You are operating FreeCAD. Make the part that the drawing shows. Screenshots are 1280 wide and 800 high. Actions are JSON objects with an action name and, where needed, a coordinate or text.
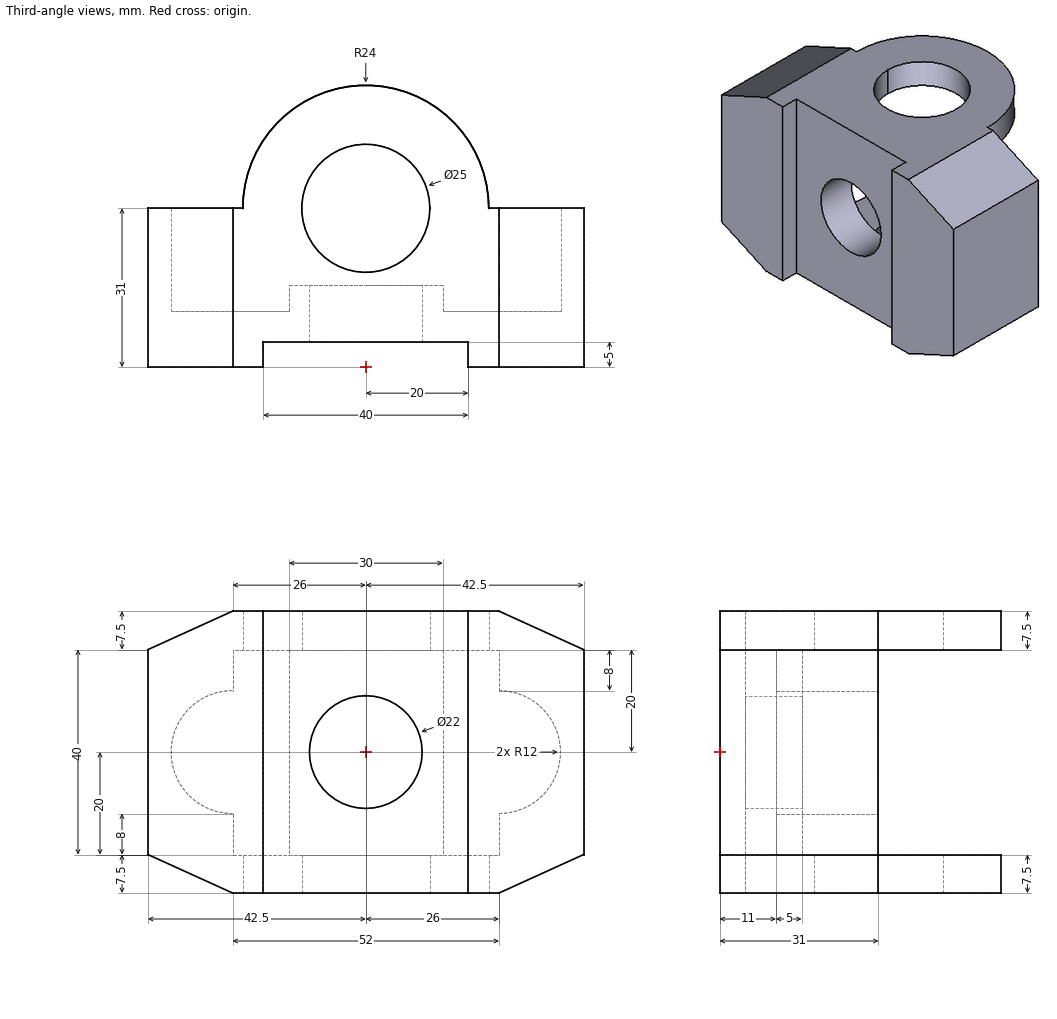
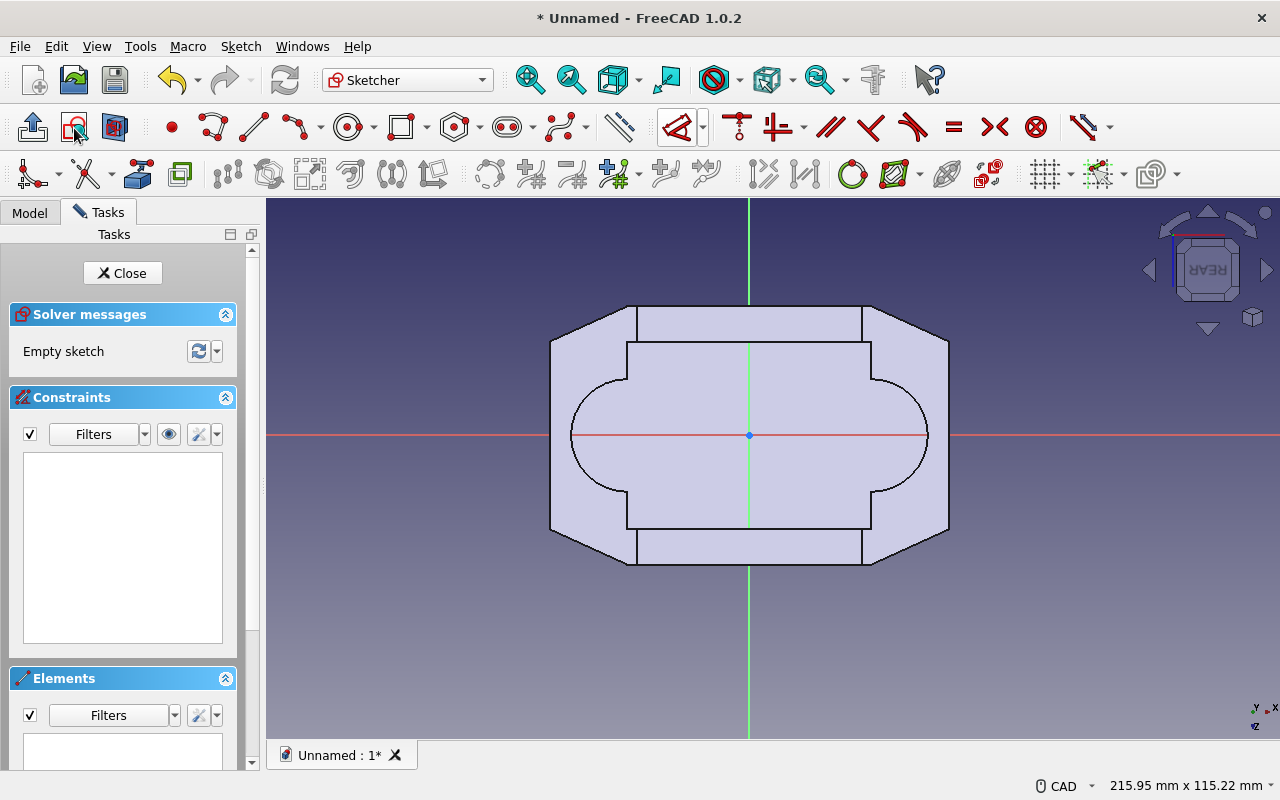
{"action": "left_click", "coordinate": [115, 128]}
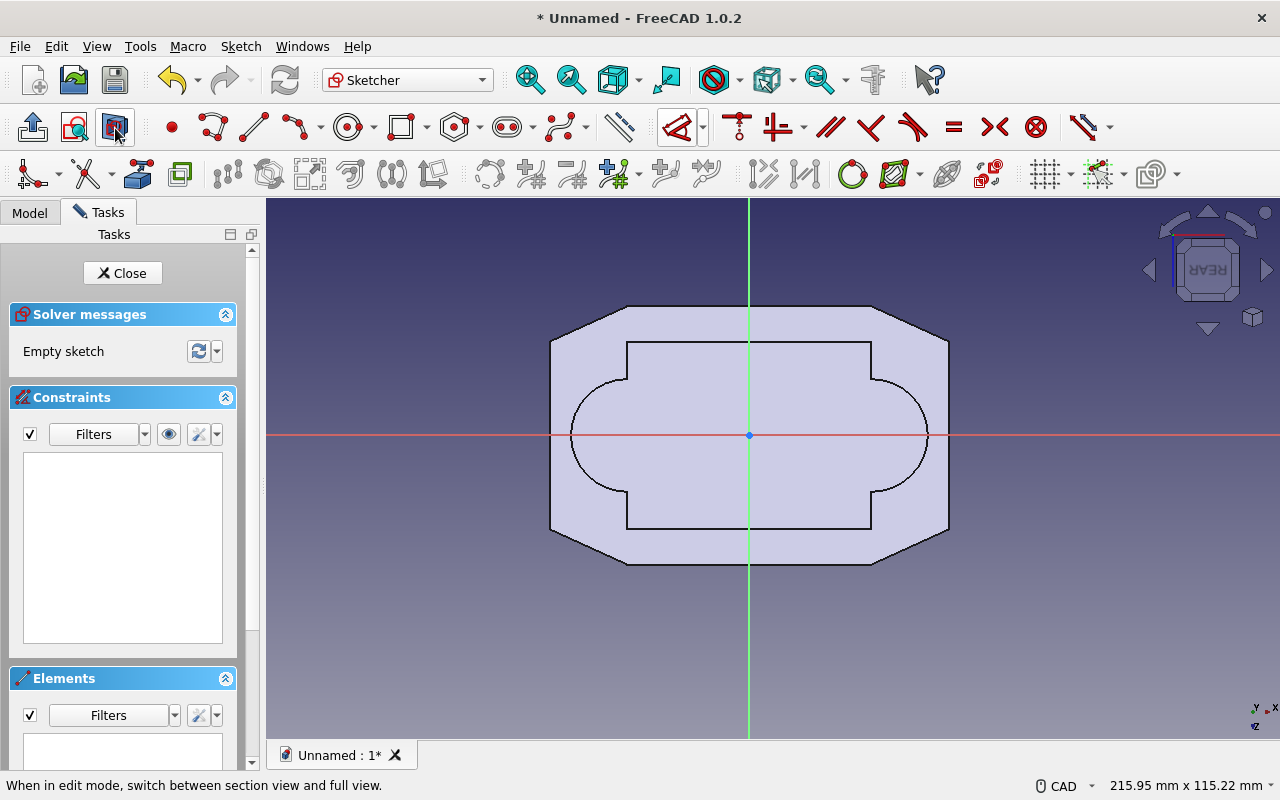
{"action": "scroll", "coordinate": [804, 395], "scroll_direction": "up", "scroll_amount": 3}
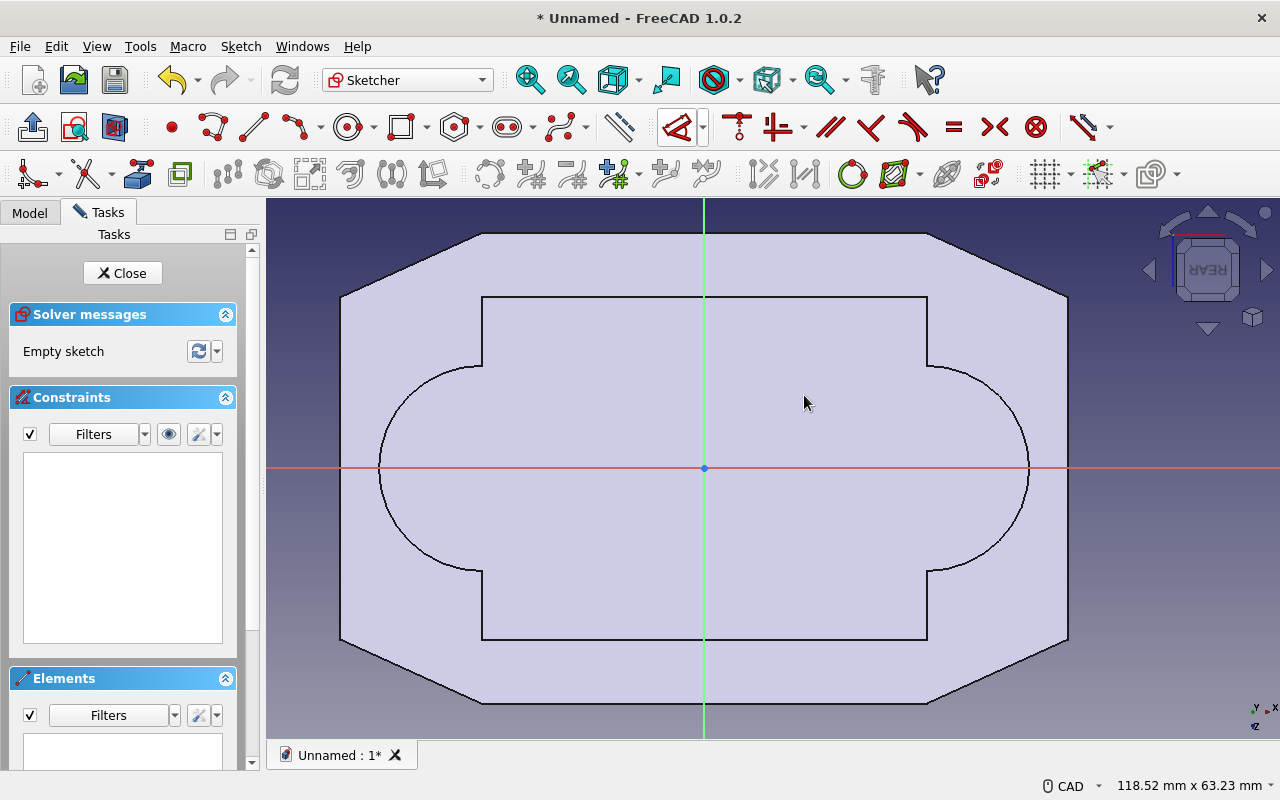
{"action": "key", "text": "g v"}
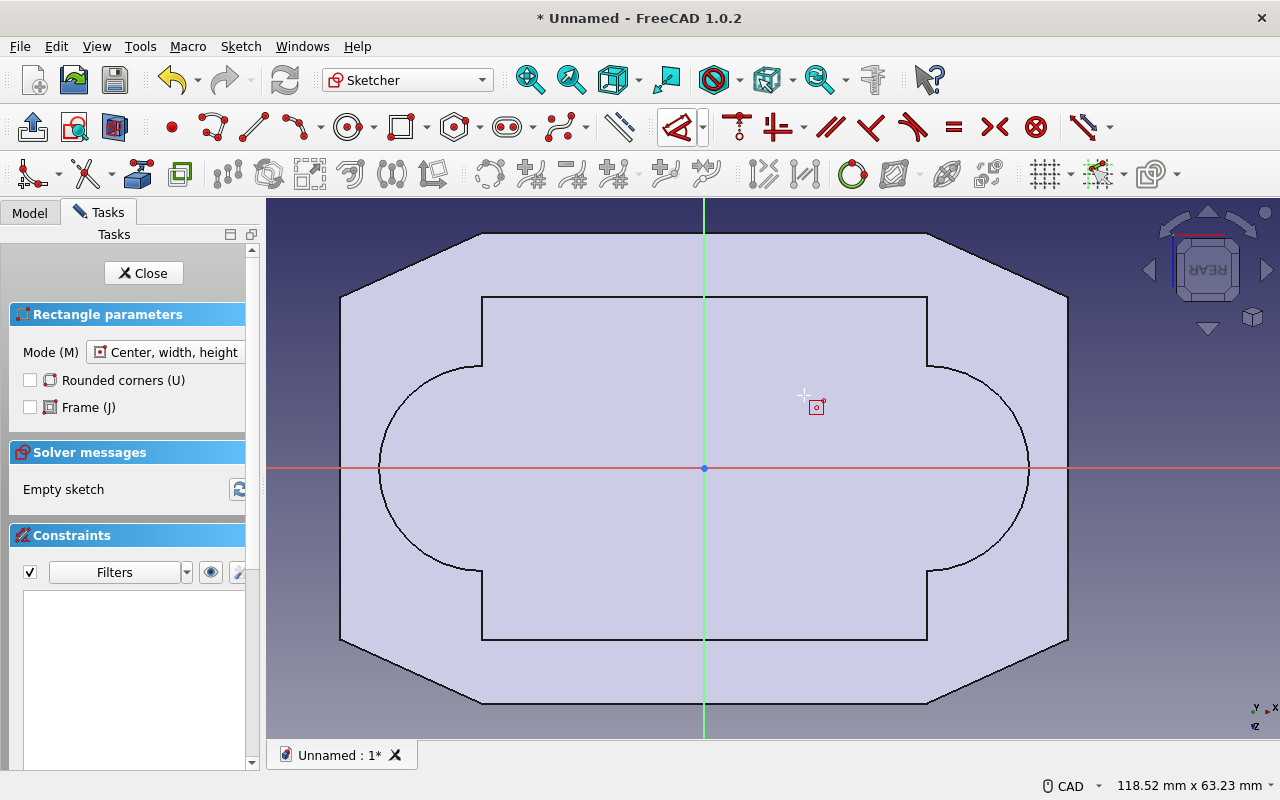
{"action": "left_click", "coordinate": [704, 468]}
{"action": "left_click", "coordinate": [832, 297]}
{"action": "key", "text": "Escape"}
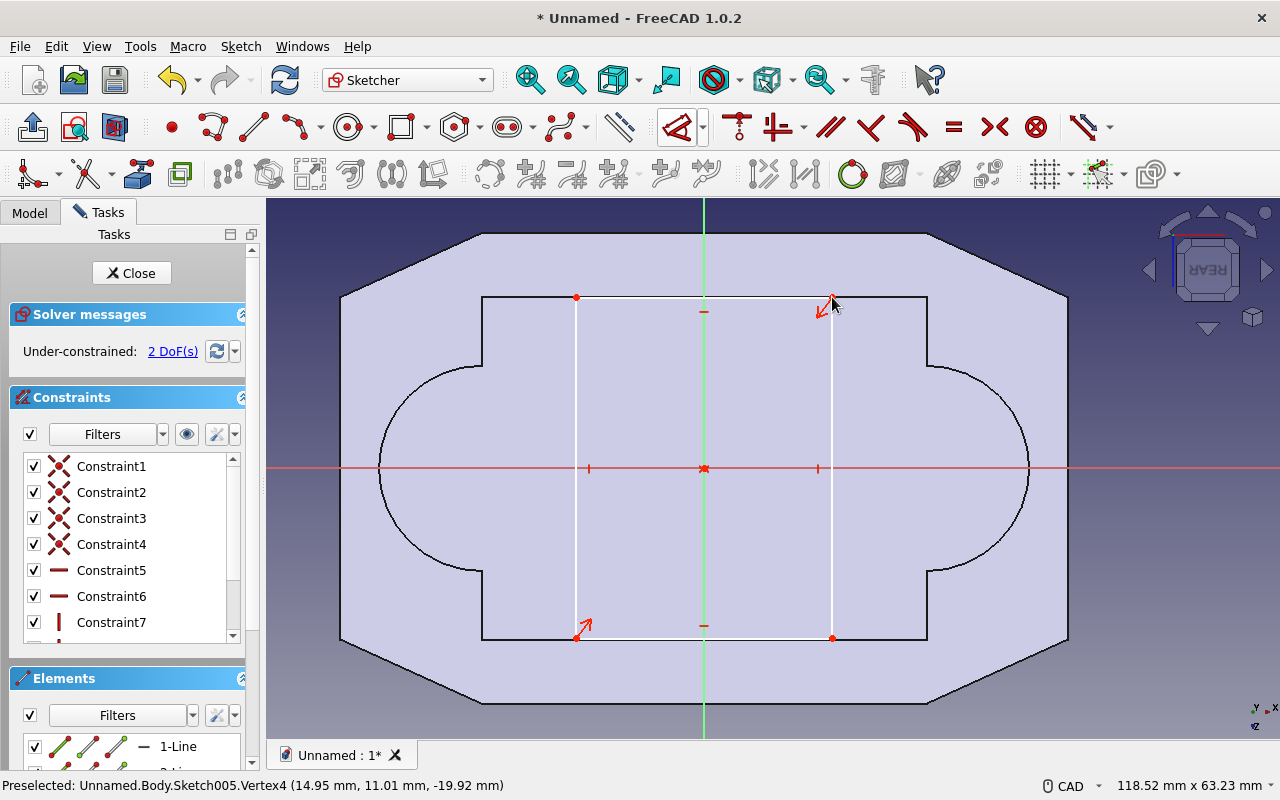
{"action": "left_click", "coordinate": [653, 639]}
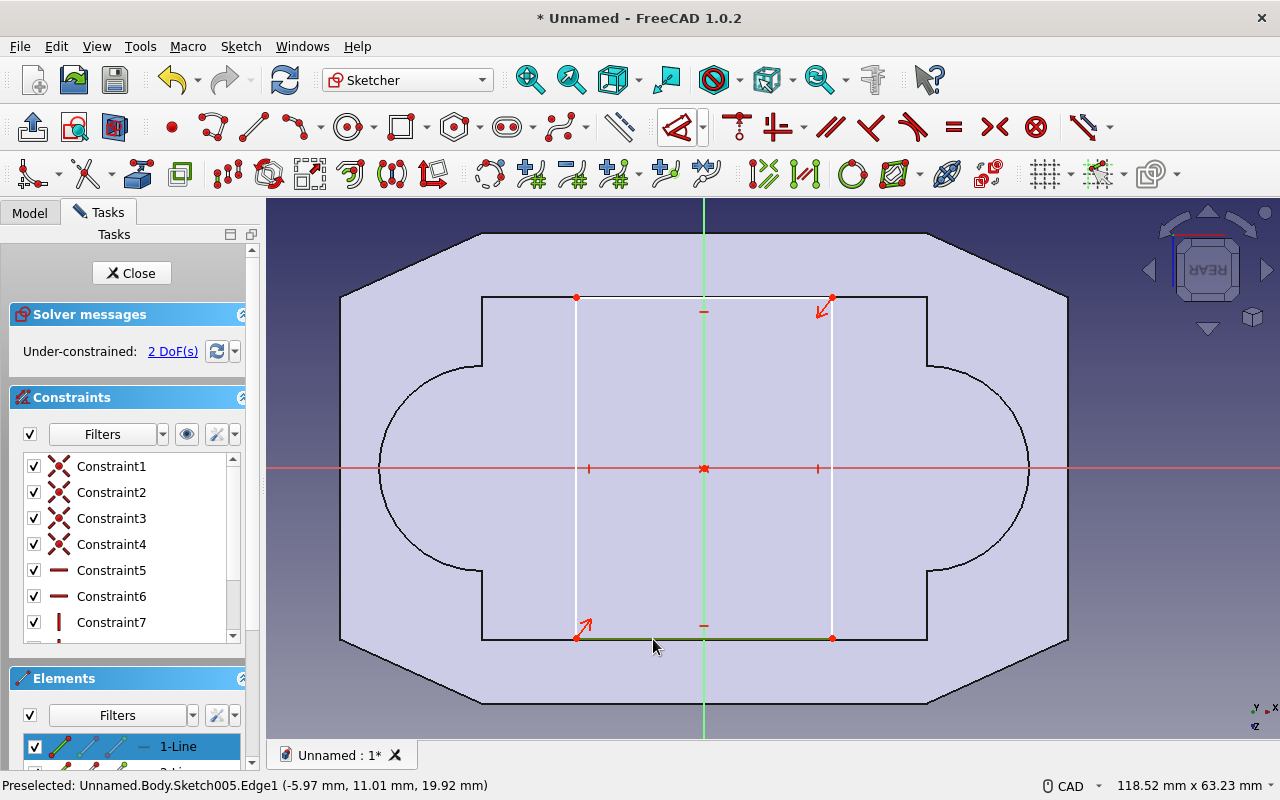
{"action": "key", "text": "l"}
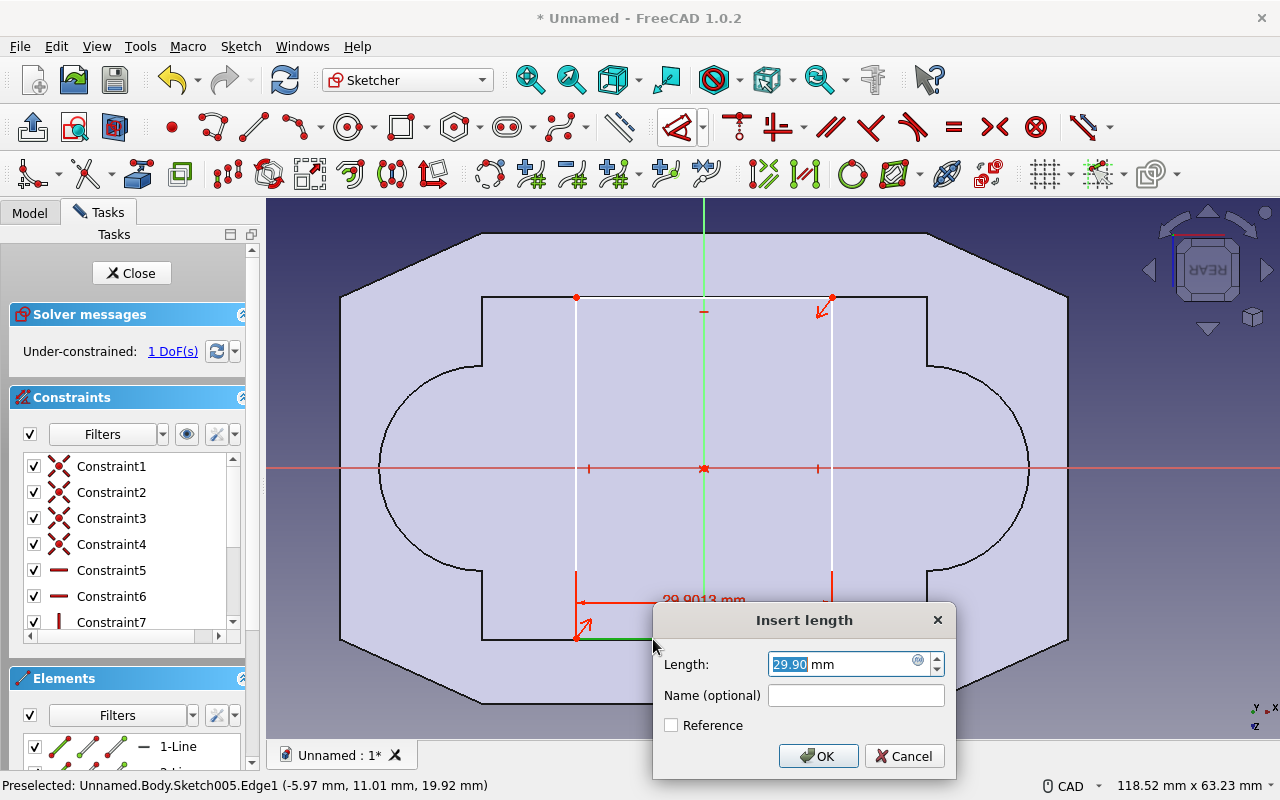
{"action": "type", "text": "30"}
{"action": "key", "text": "Return"}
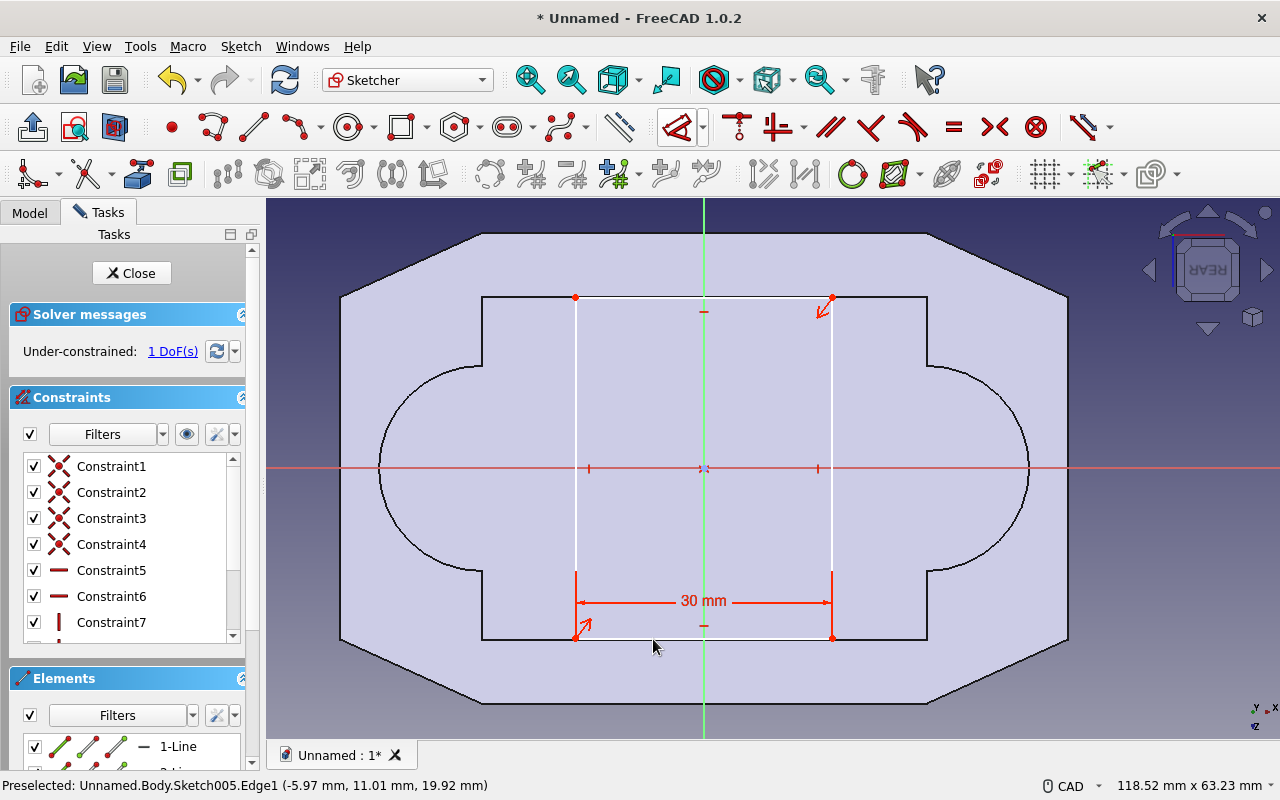
{"action": "left_click", "coordinate": [832, 537]}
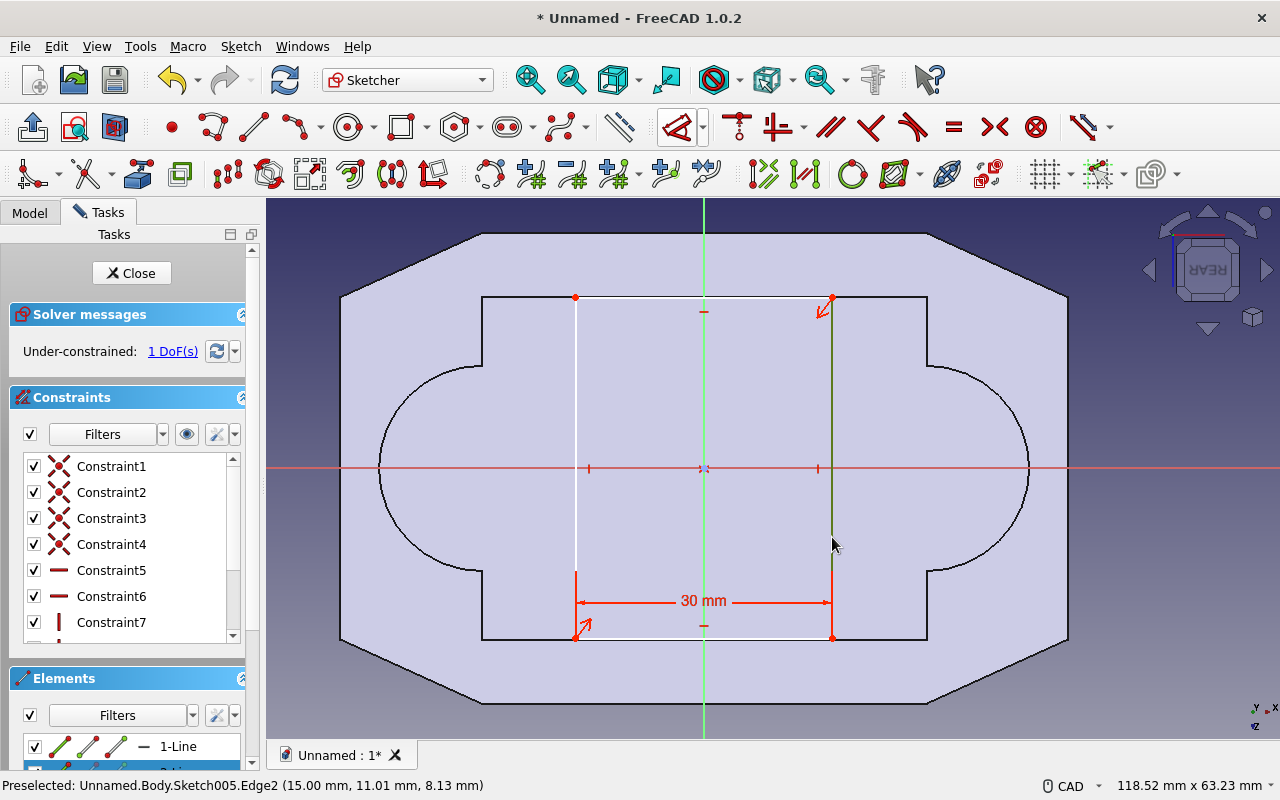
{"action": "left_click", "coordinate": [702, 128]}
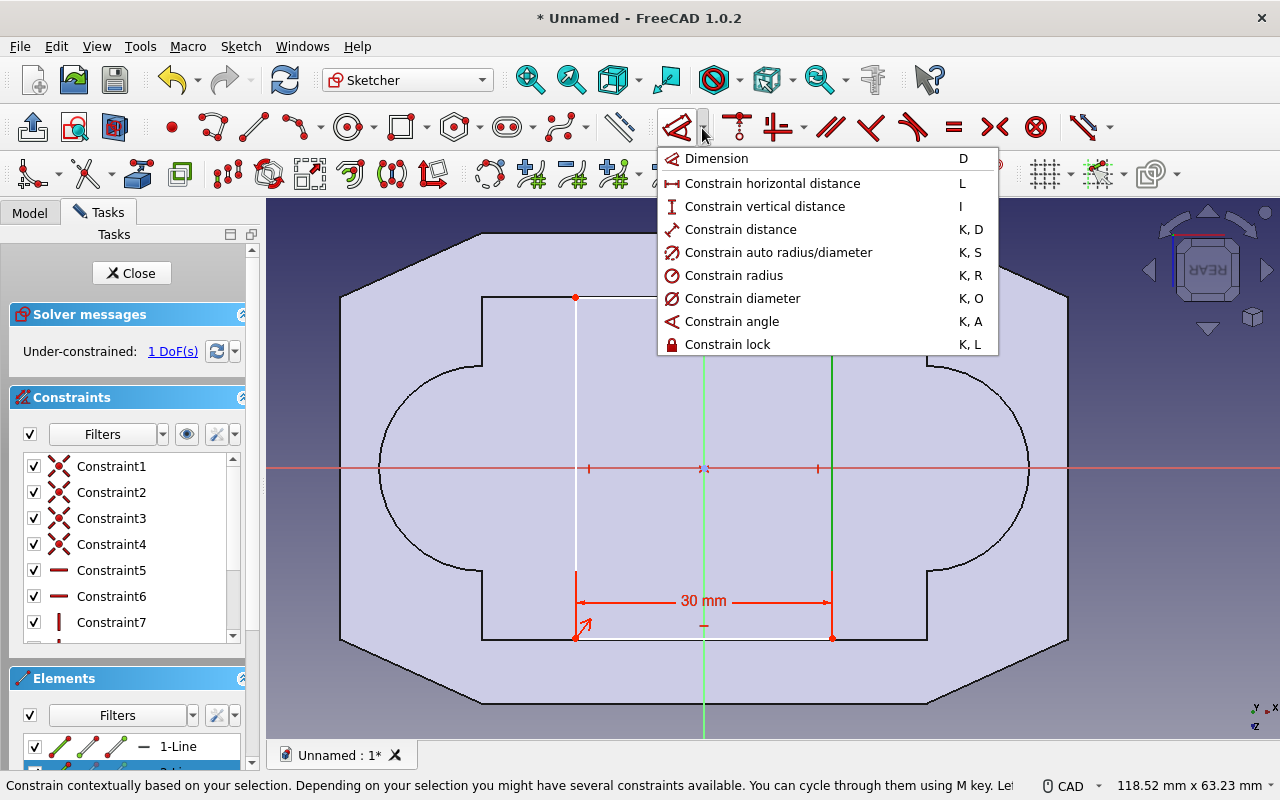
{"action": "left_click", "coordinate": [828, 206]}